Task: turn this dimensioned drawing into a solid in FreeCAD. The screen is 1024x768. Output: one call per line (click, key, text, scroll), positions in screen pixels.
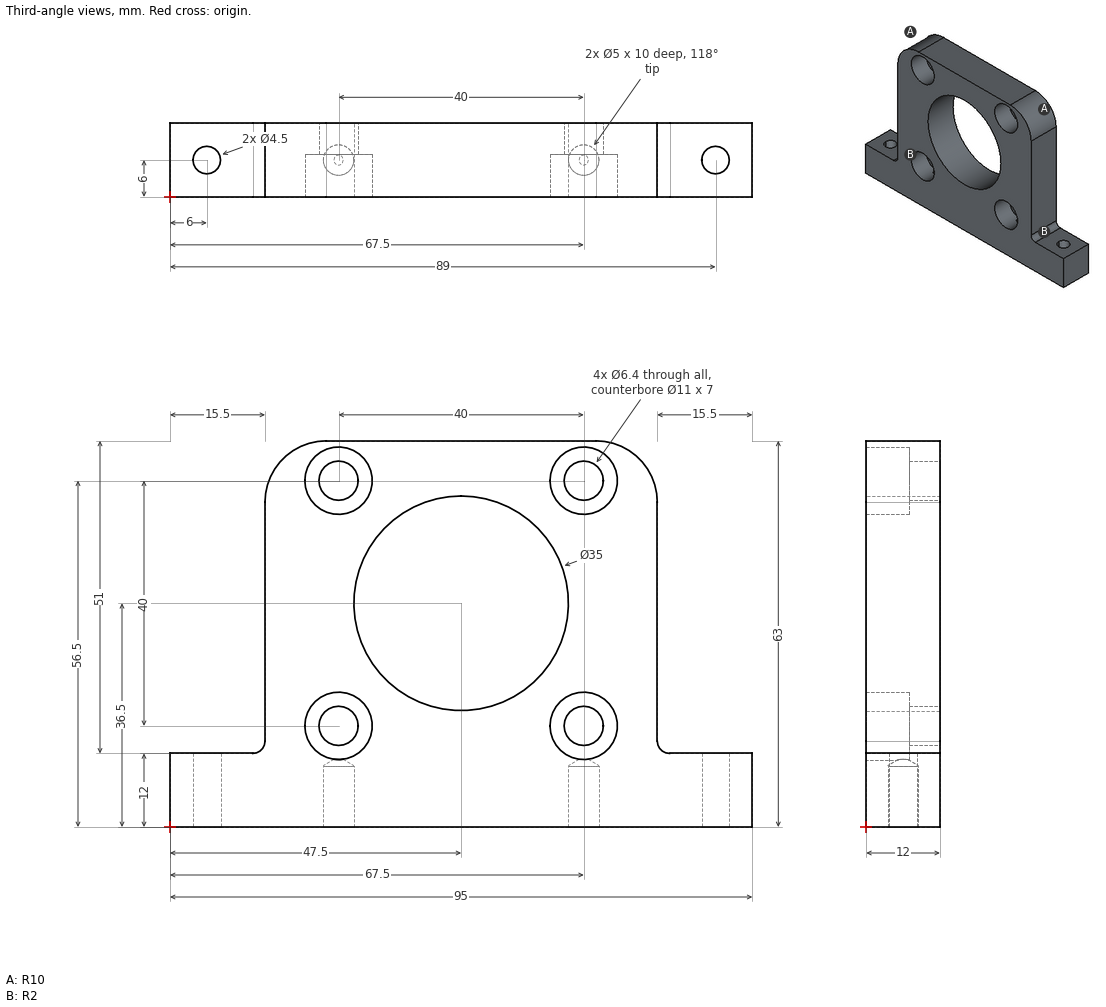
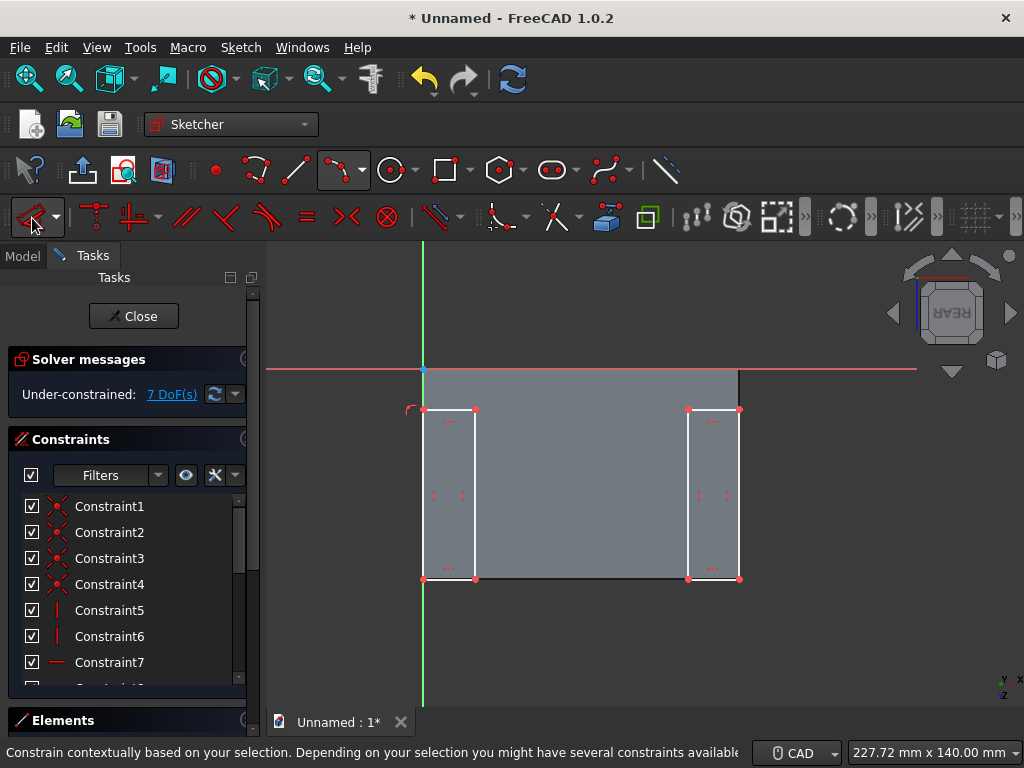
click(423, 461)
click(389, 495)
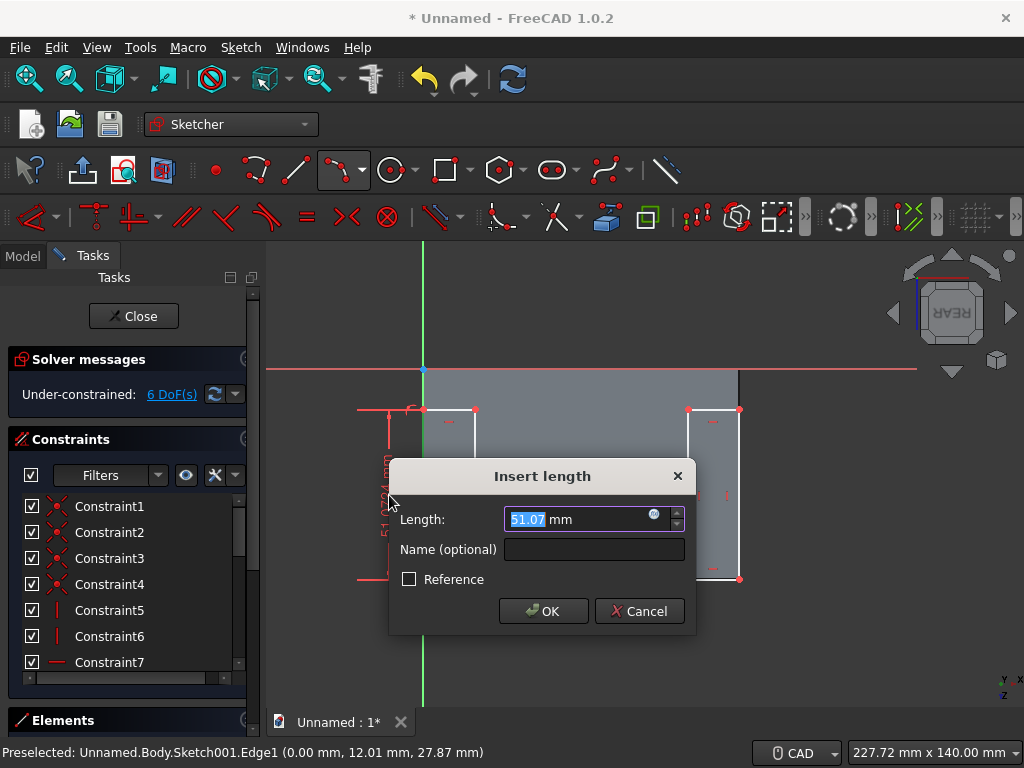
text(51)
key(Return)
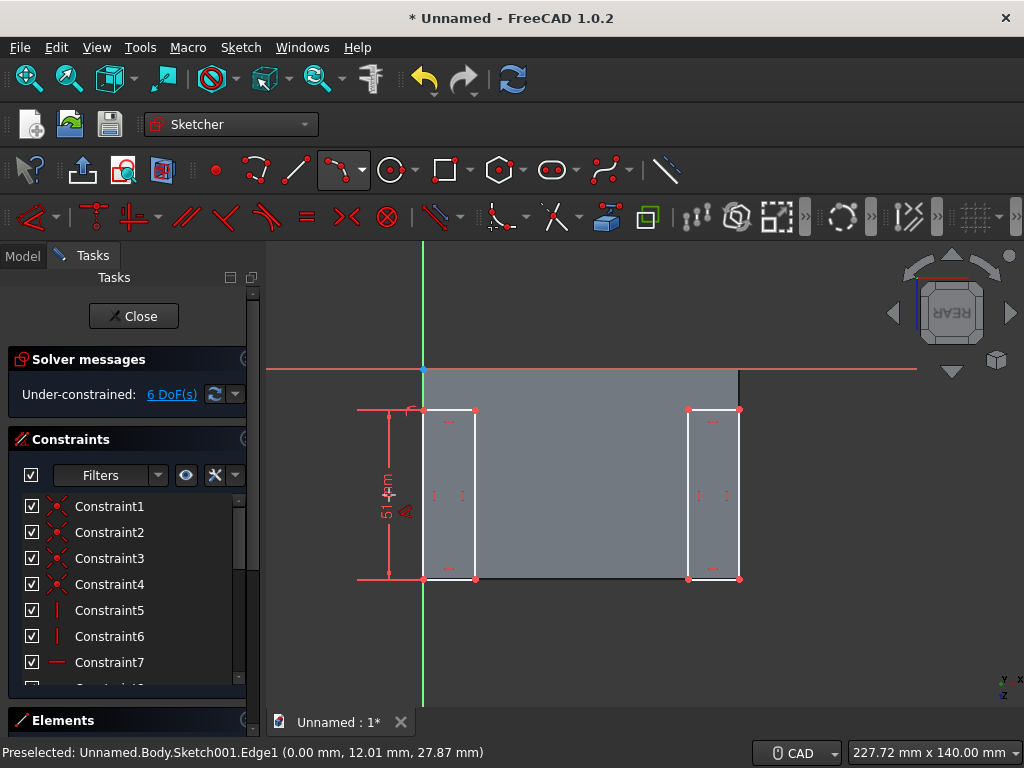
click(688, 461)
click(722, 495)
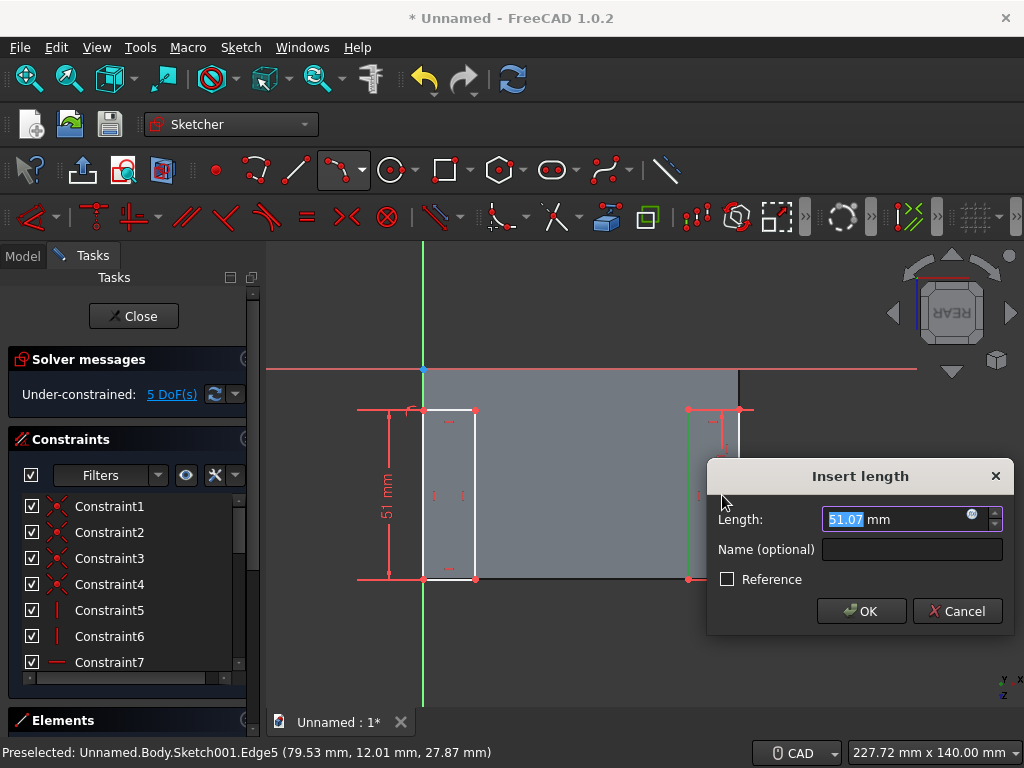
text(51)
key(Return)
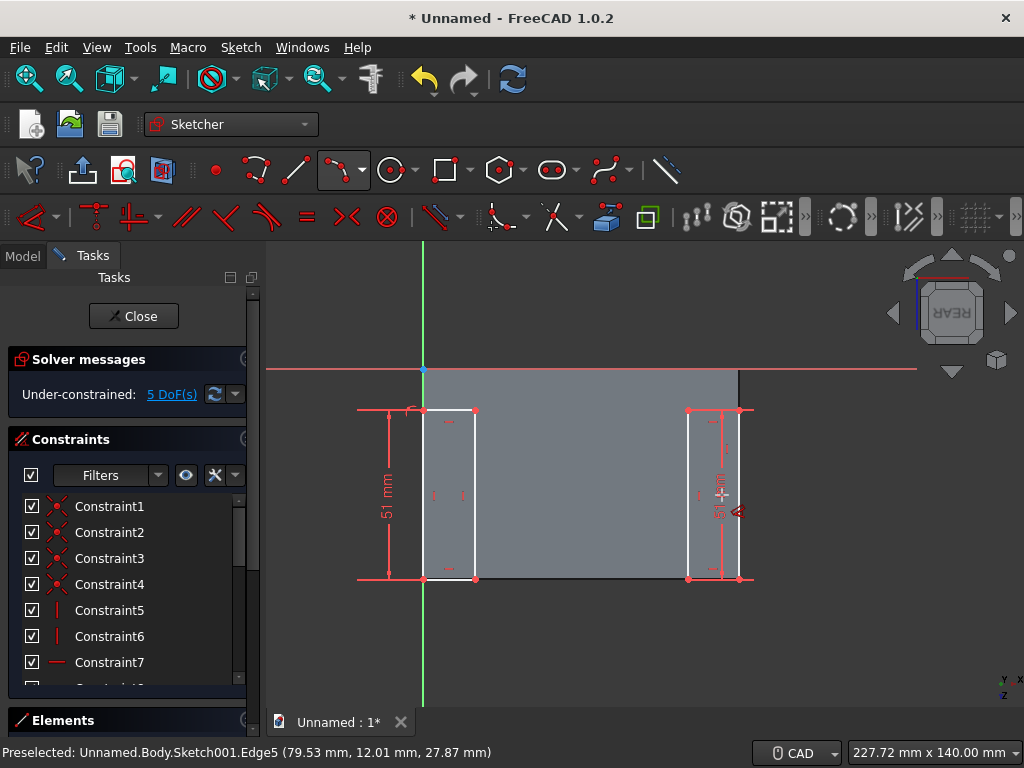
click(423, 410)
click(389, 390)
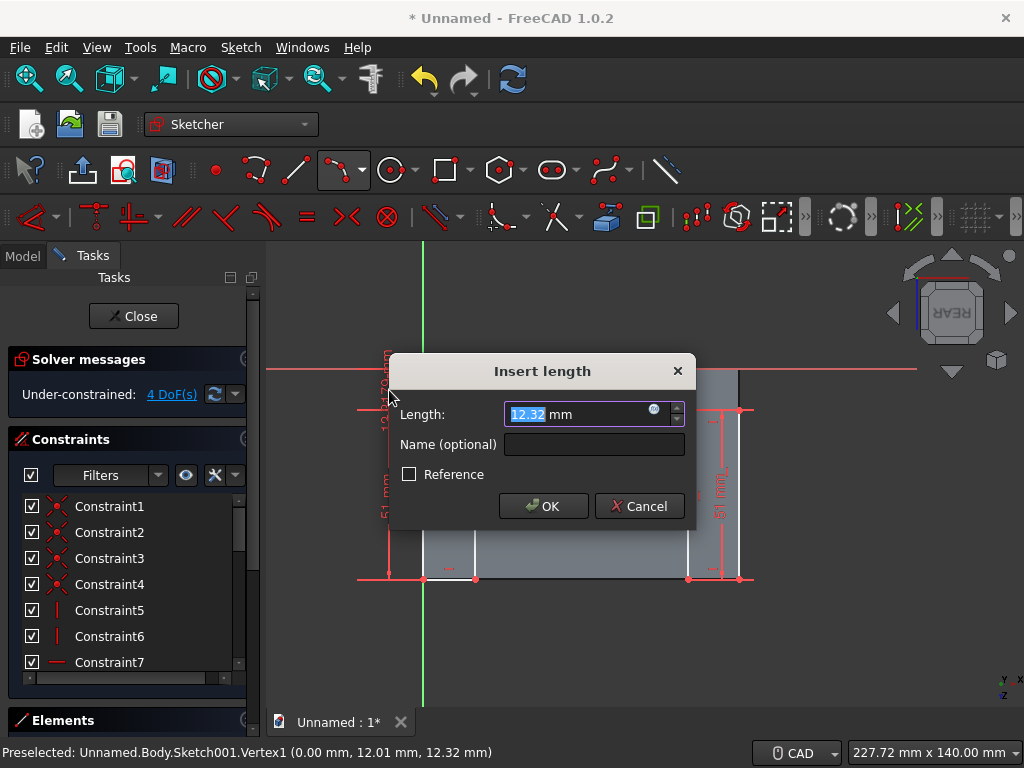
text(12)
key(Return)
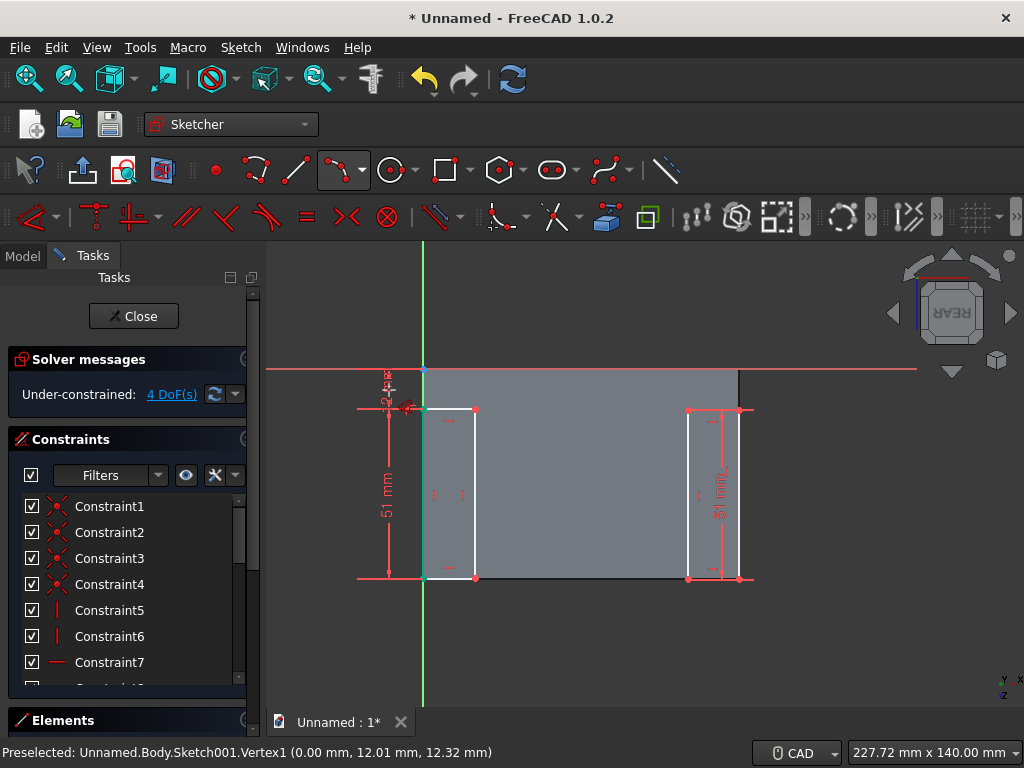
click(688, 410)
click(722, 390)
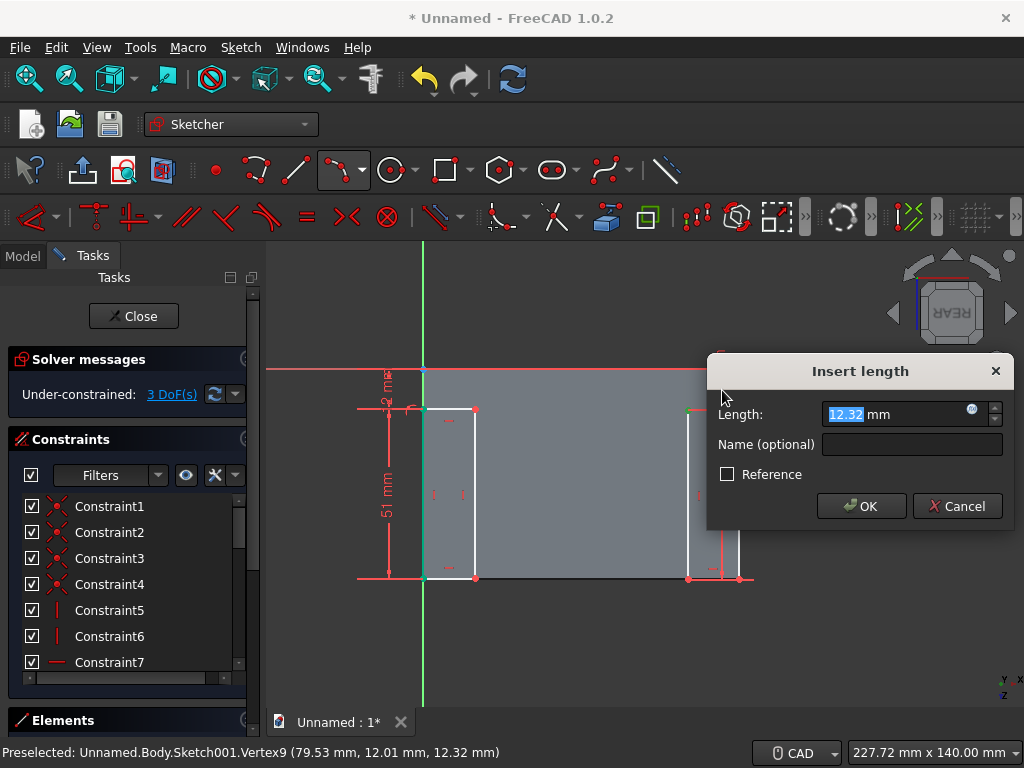
text(12)
key(Return)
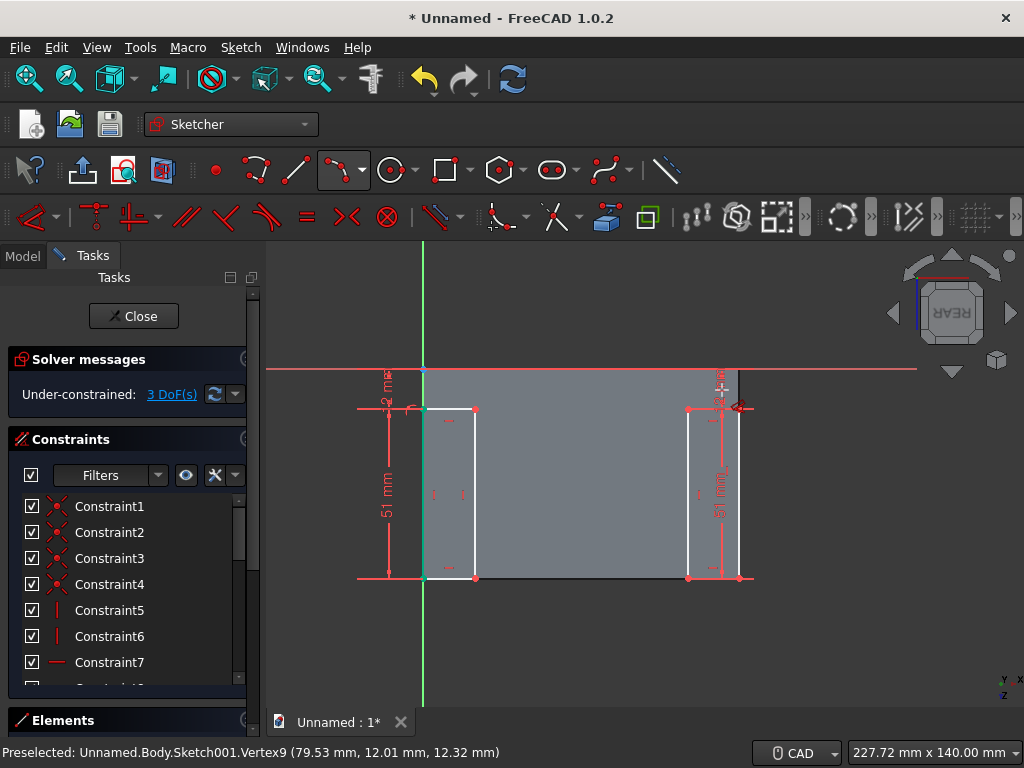
click(739, 579)
click(581, 613)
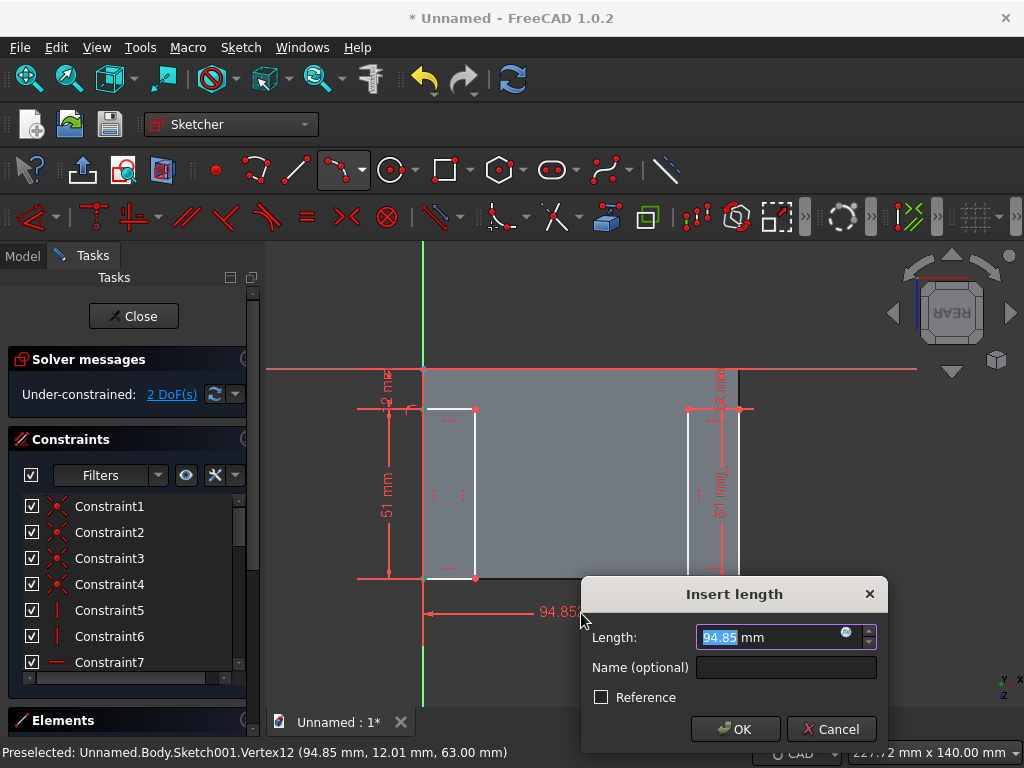
text(95)
key(Return)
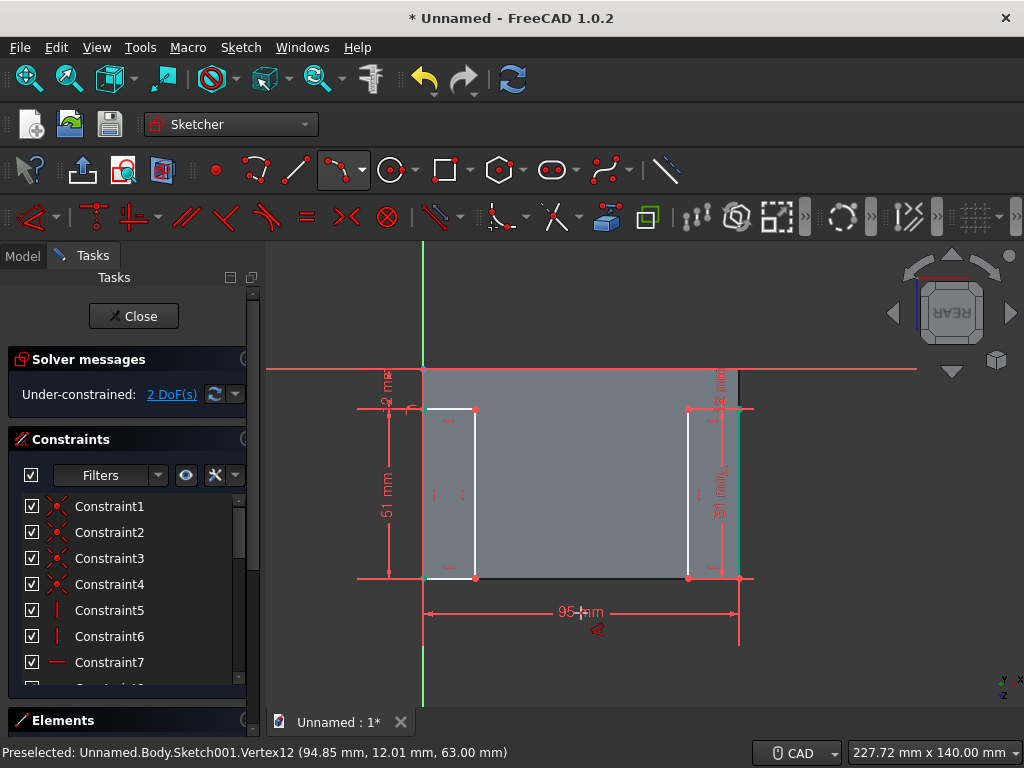
click(439, 579)
click(449, 613)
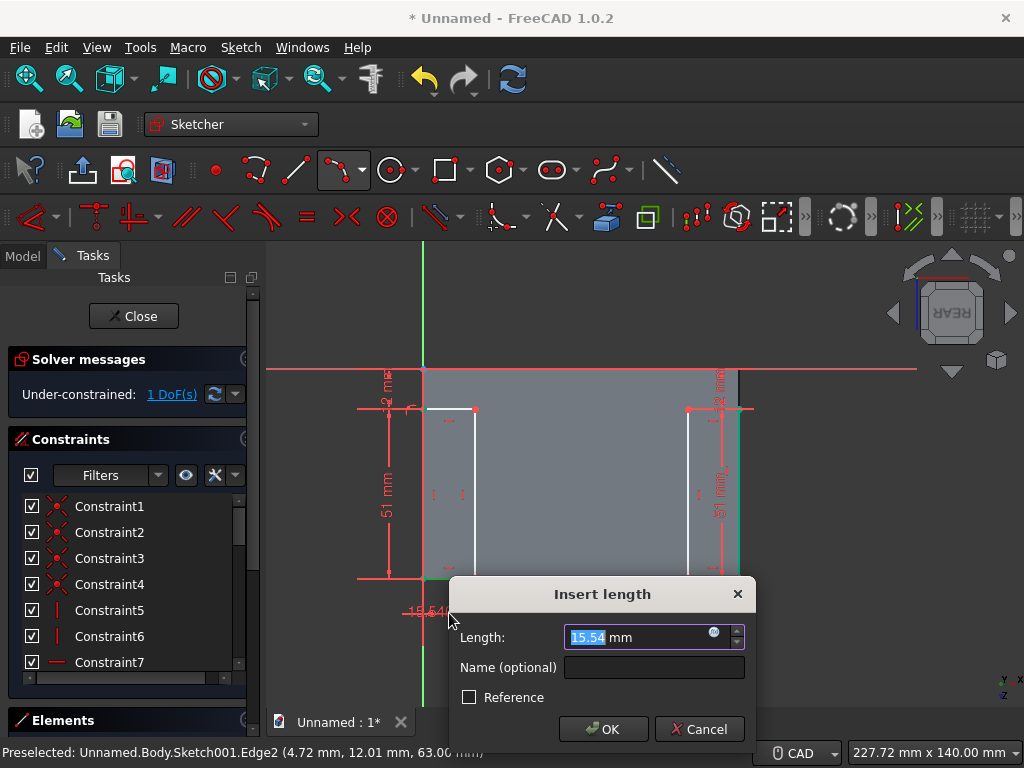
text(15.5)
key(Return)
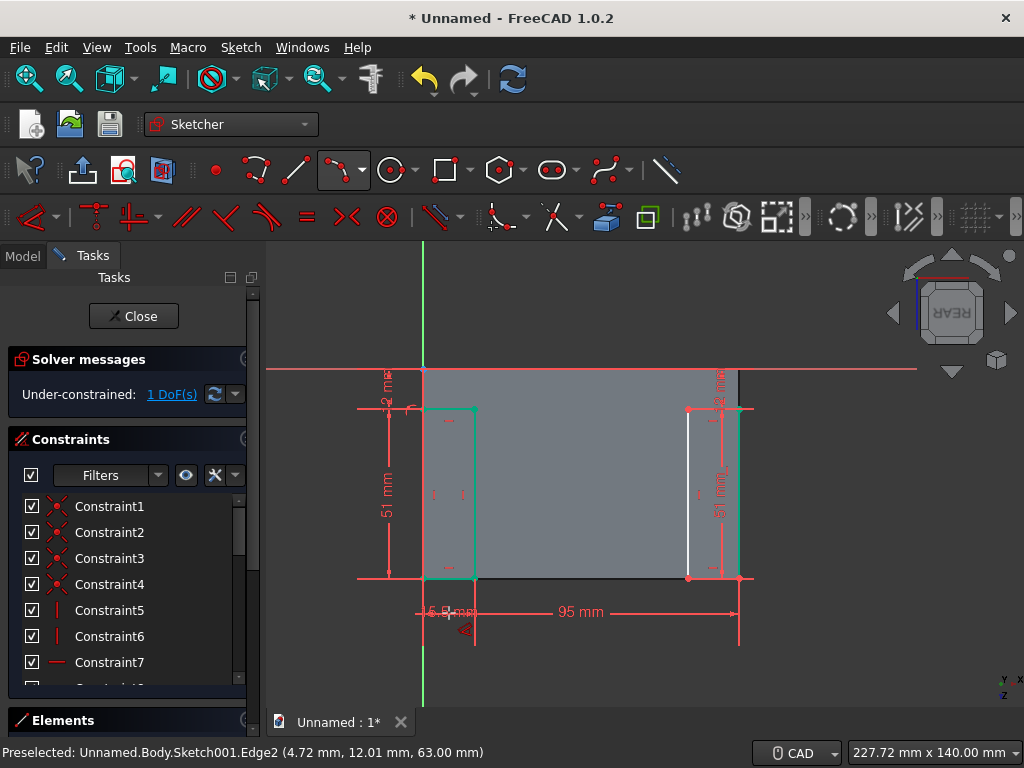
click(703, 579)
click(714, 613)